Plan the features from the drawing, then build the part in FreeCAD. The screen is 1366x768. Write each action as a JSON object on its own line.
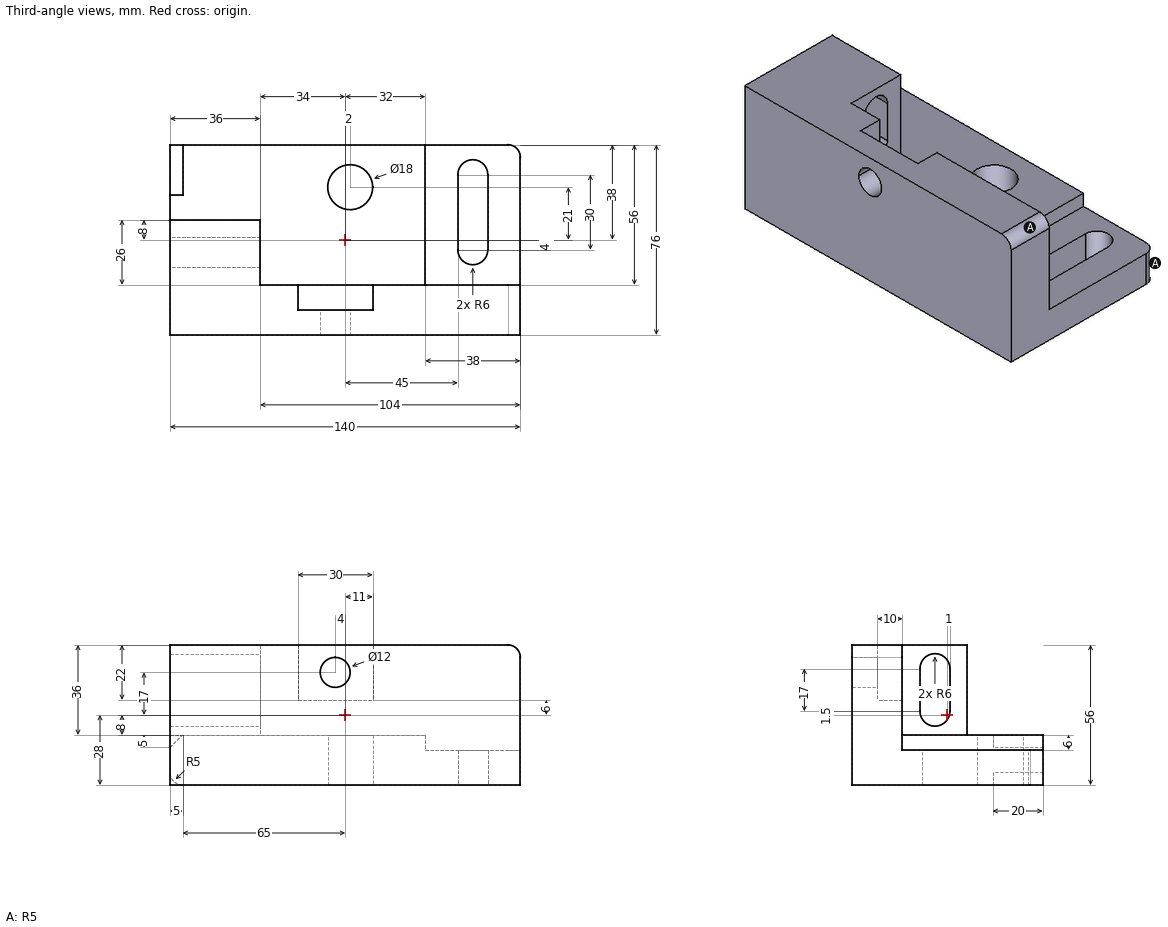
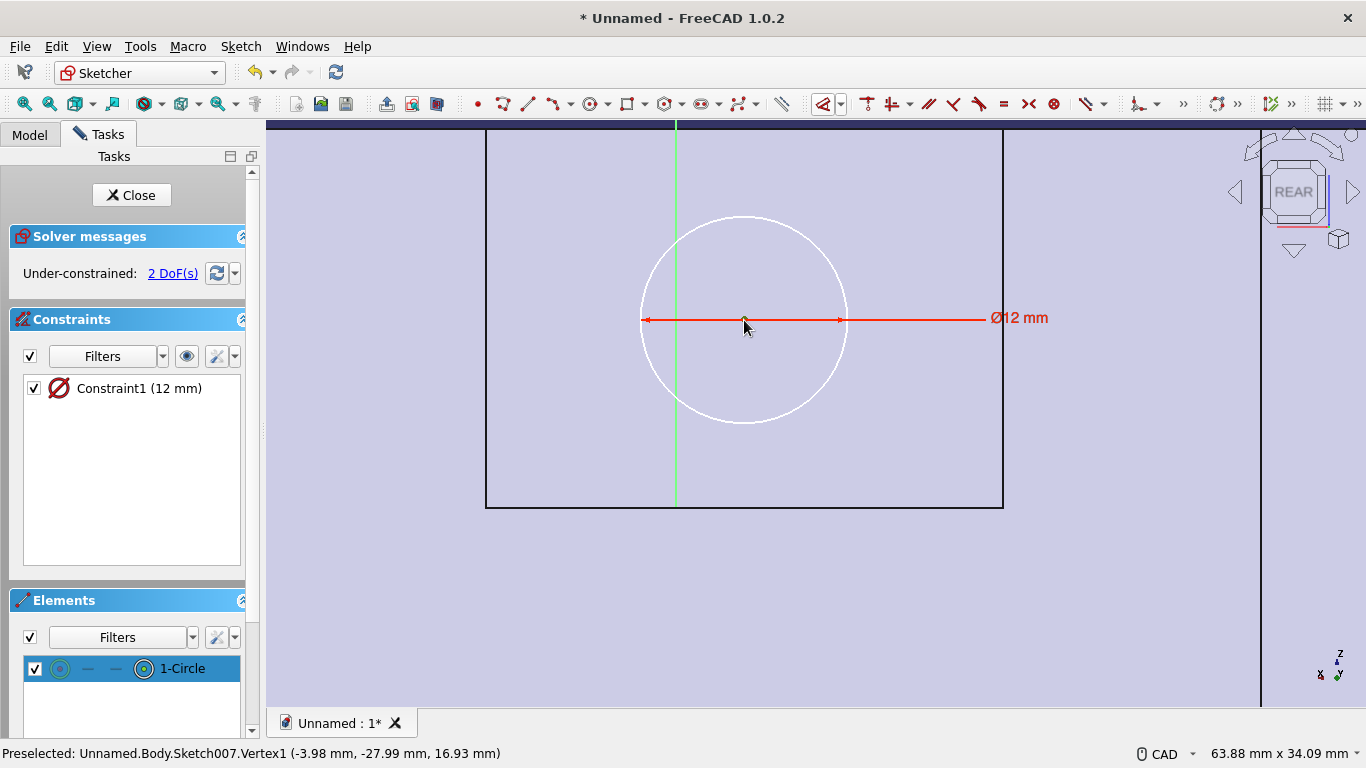
{"action": "left_click", "coordinate": [840, 104]}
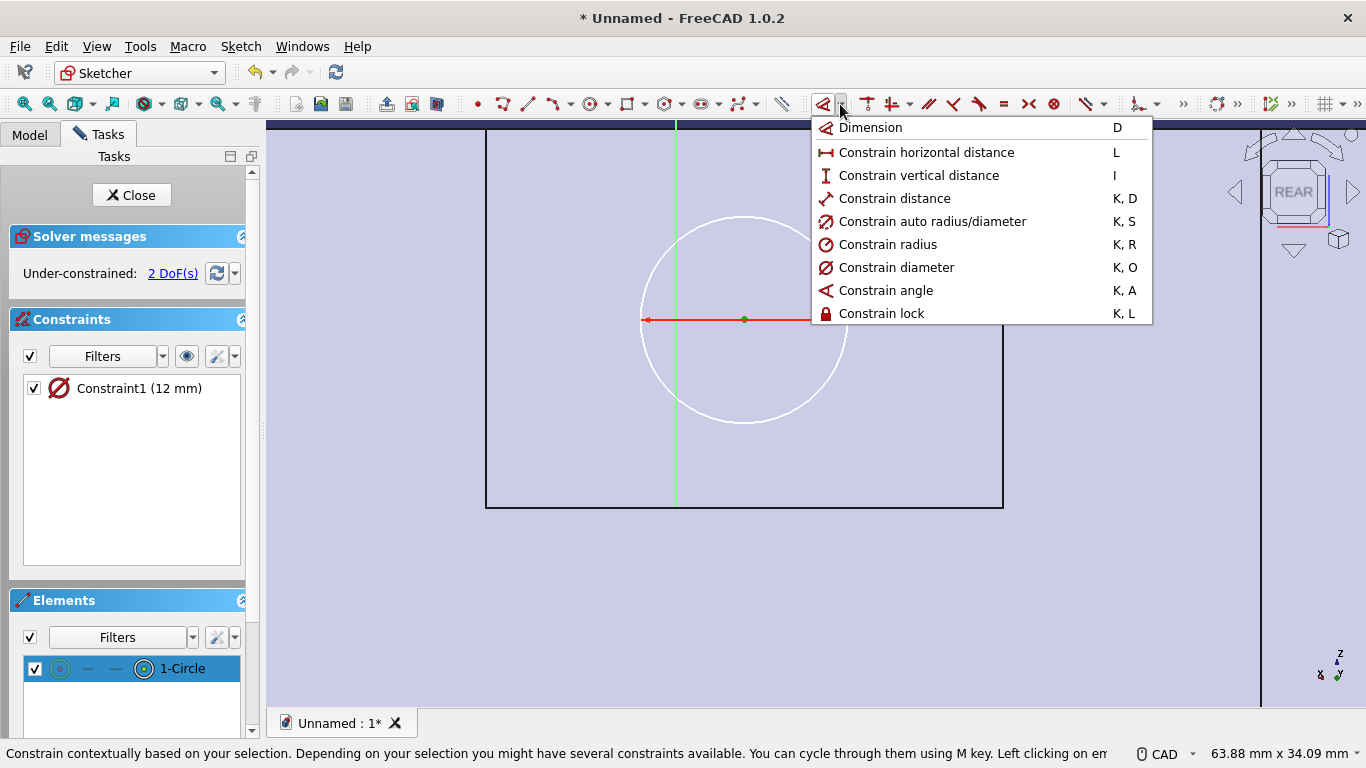
{"action": "left_click", "coordinate": [982, 152]}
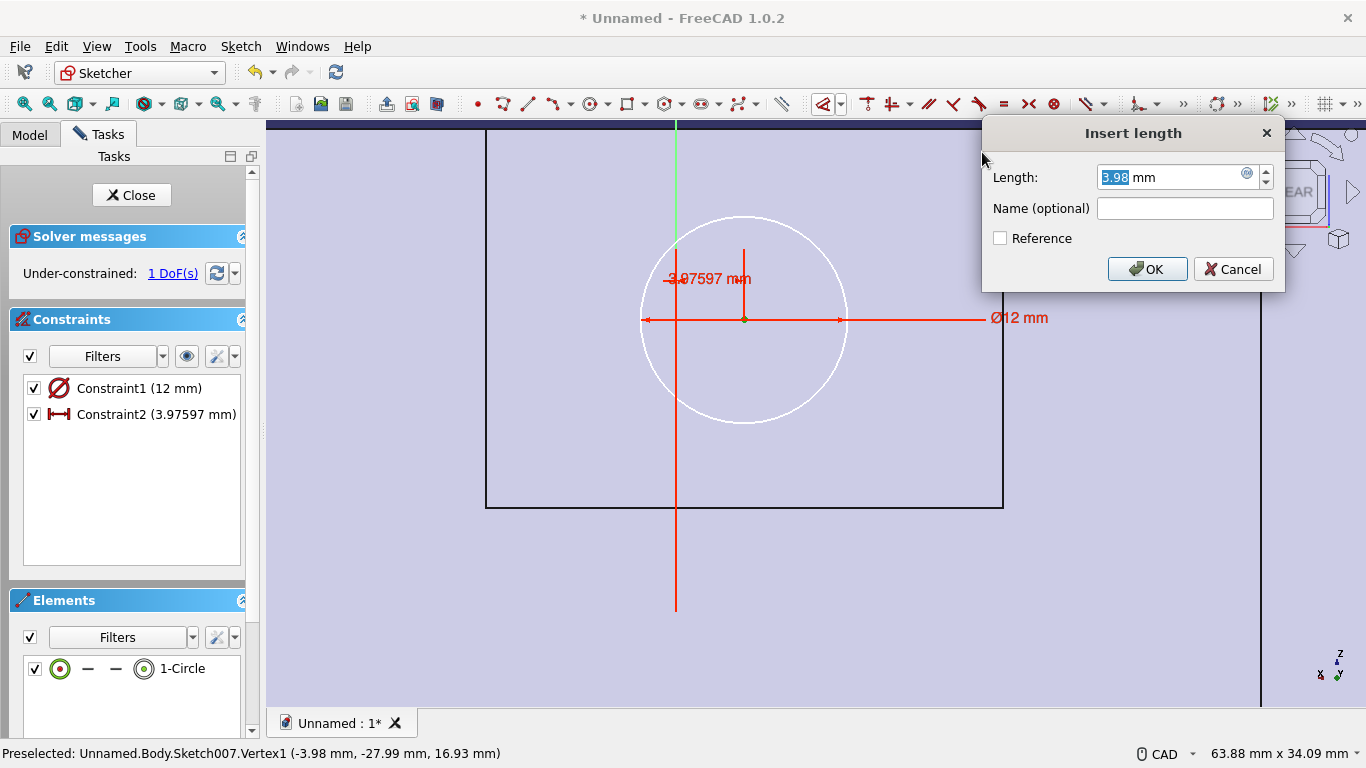
{"action": "type", "text": "4"}
{"action": "key", "text": "Return"}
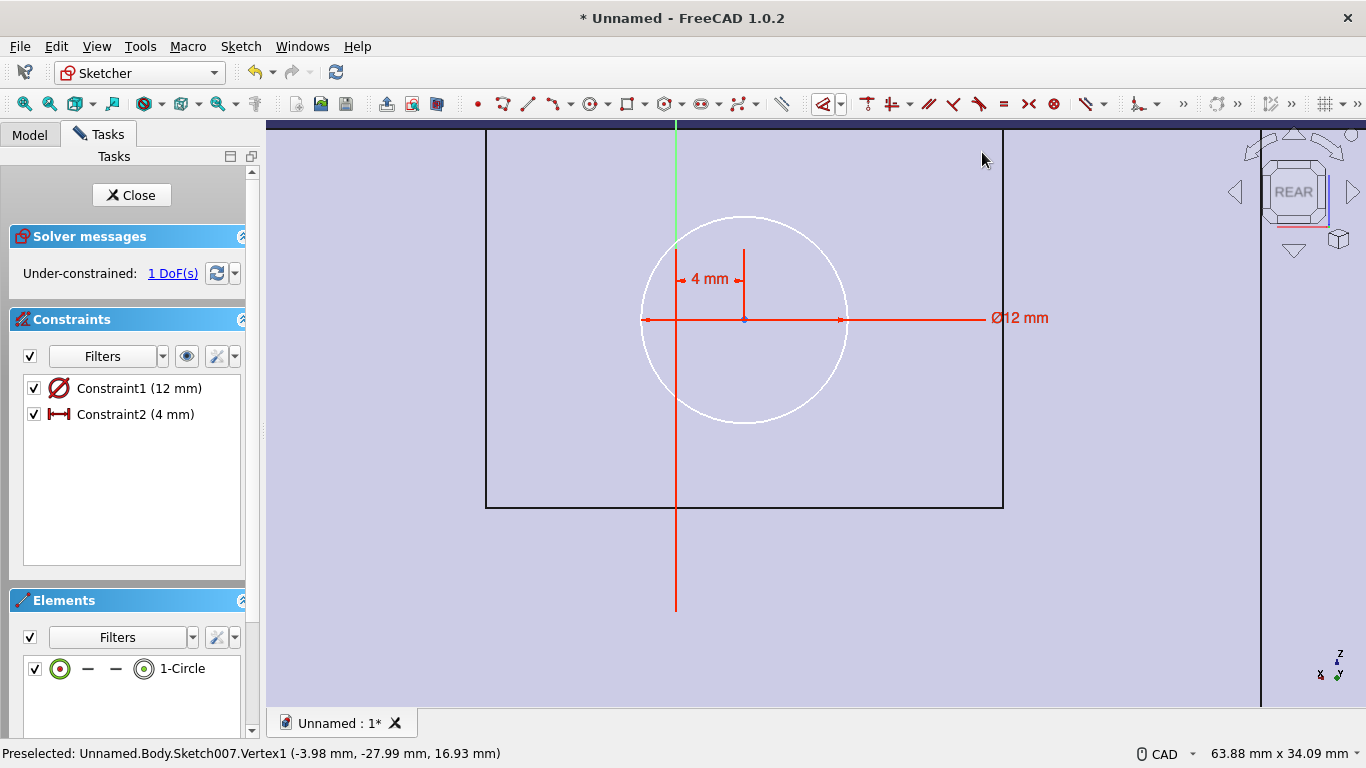
{"action": "left_click", "coordinate": [744, 320]}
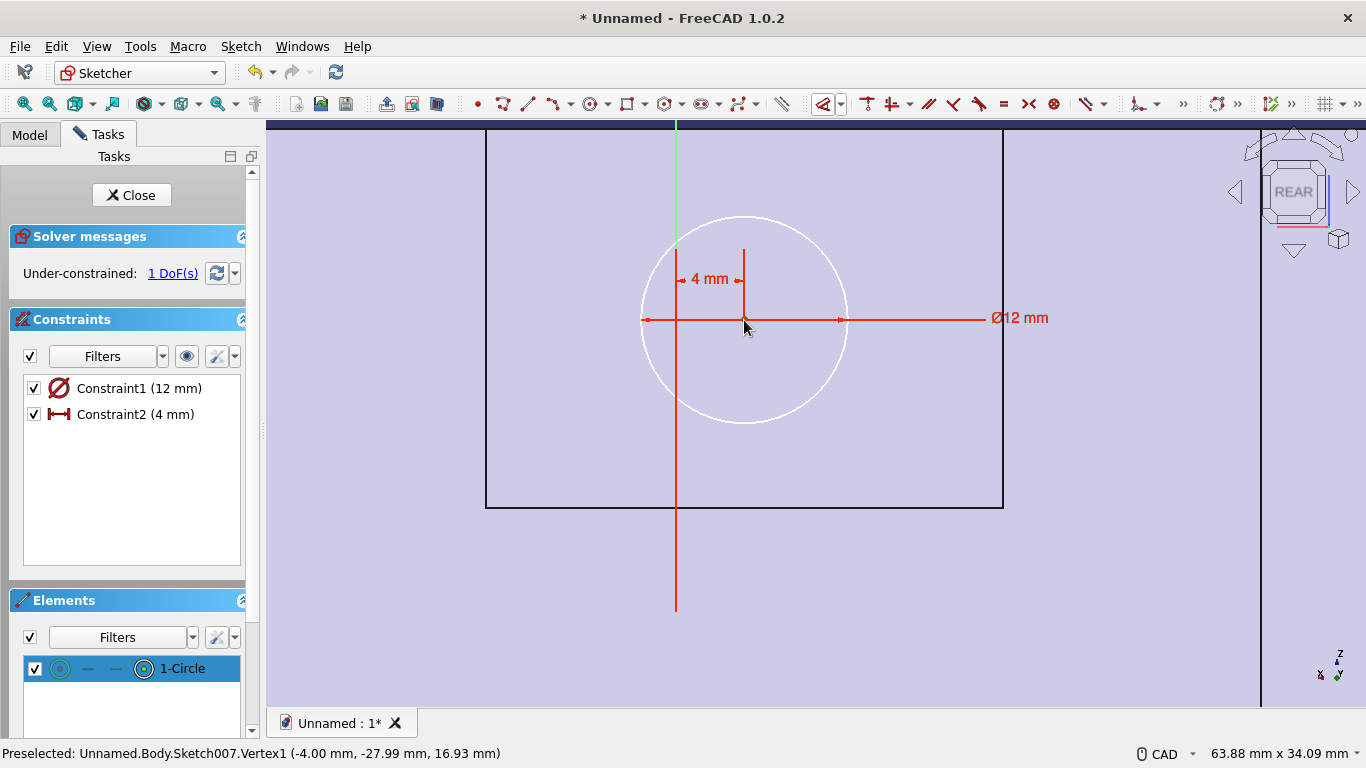
{"action": "left_click", "coordinate": [840, 104]}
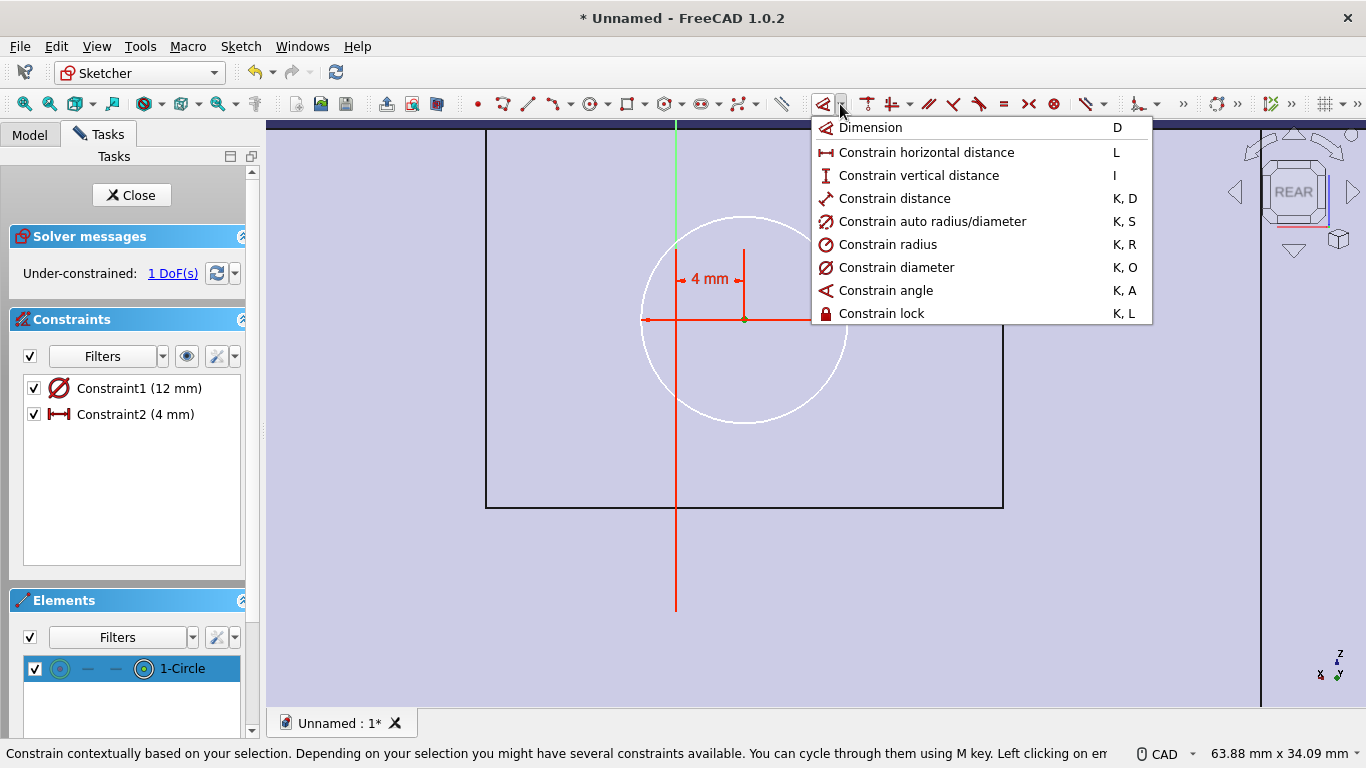
{"action": "left_click", "coordinate": [982, 176]}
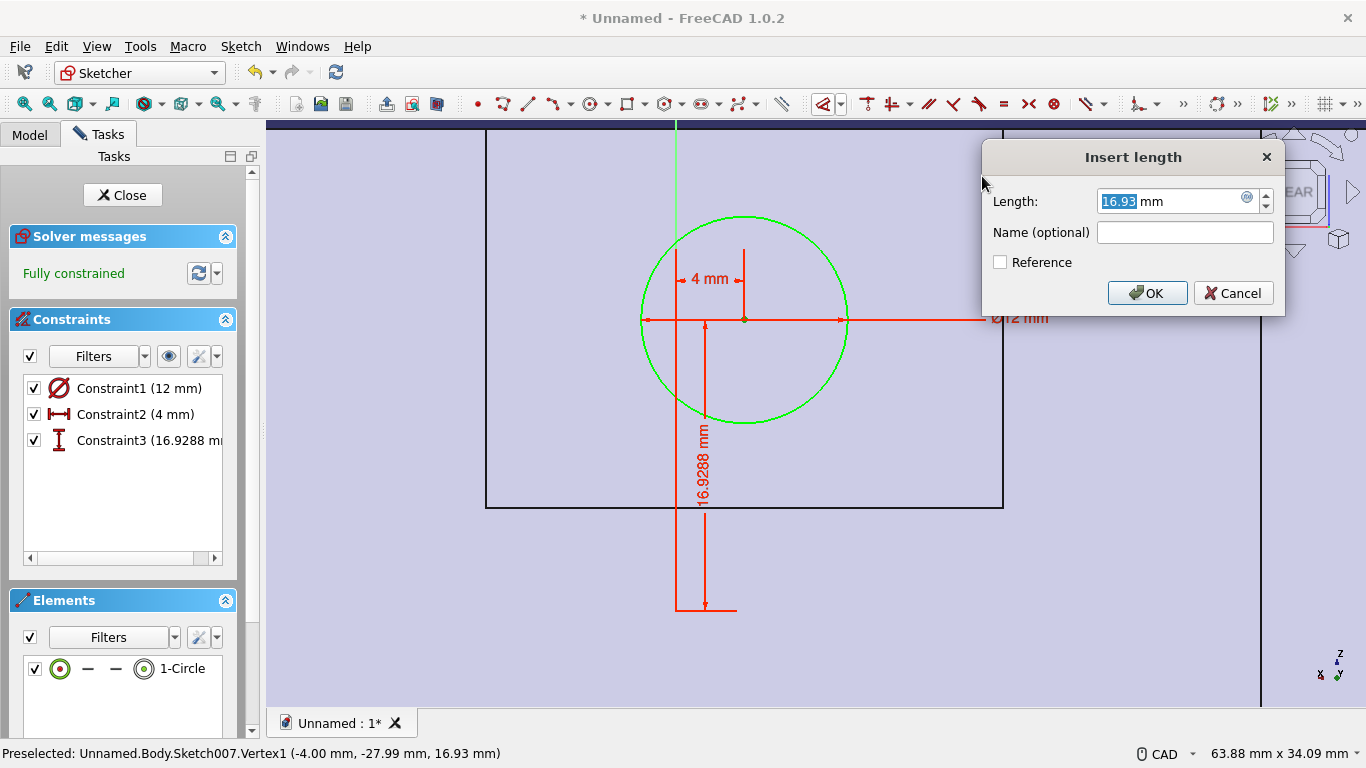
{"action": "type", "text": "17"}
{"action": "key", "text": "Return"}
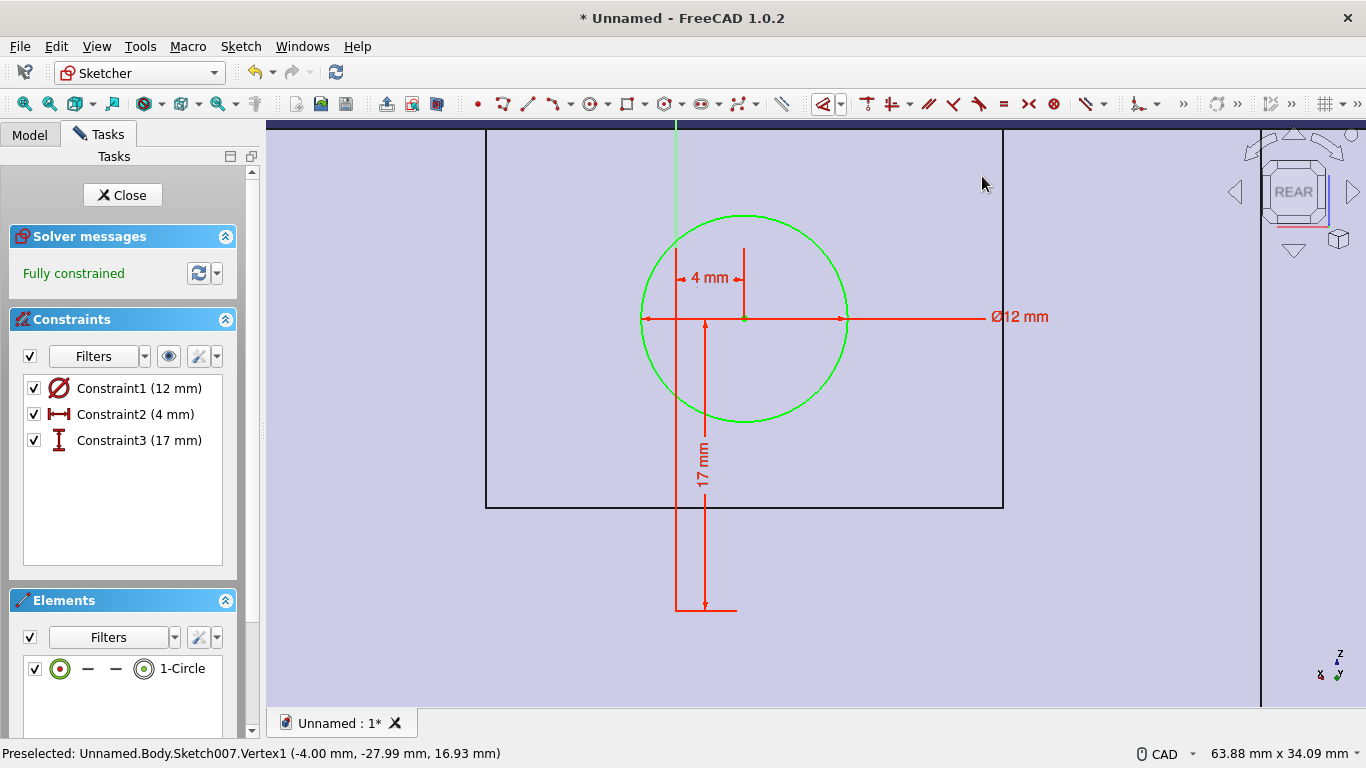
{"action": "left_click", "coordinate": [123, 195]}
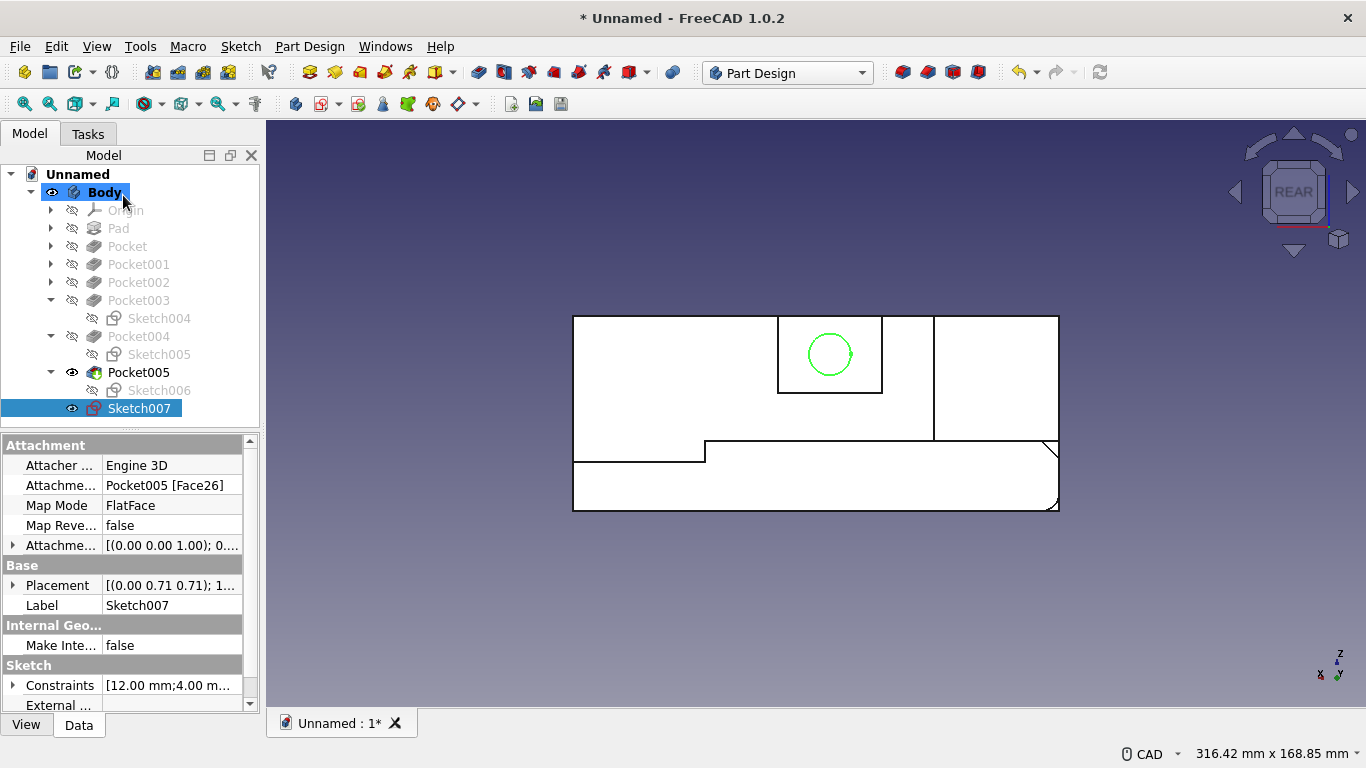
{"action": "left_click", "coordinate": [479, 72]}